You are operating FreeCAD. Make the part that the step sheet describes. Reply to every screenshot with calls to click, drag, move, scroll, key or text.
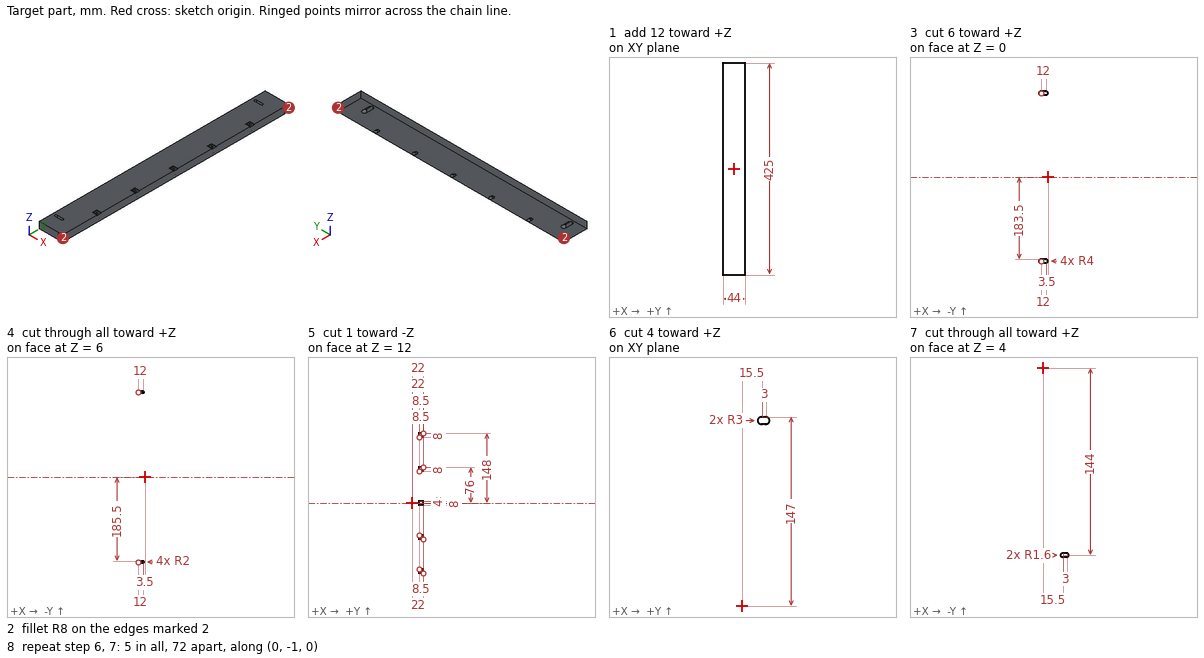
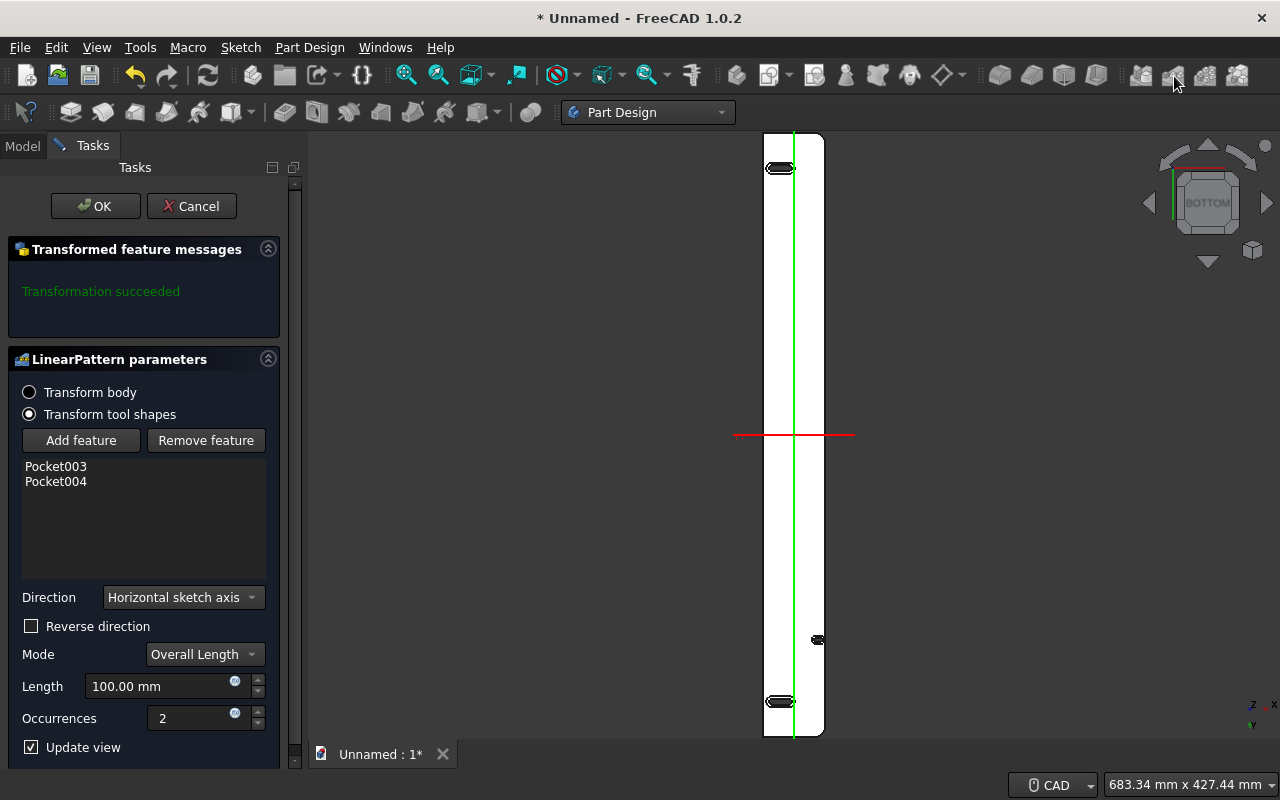
click(184, 598)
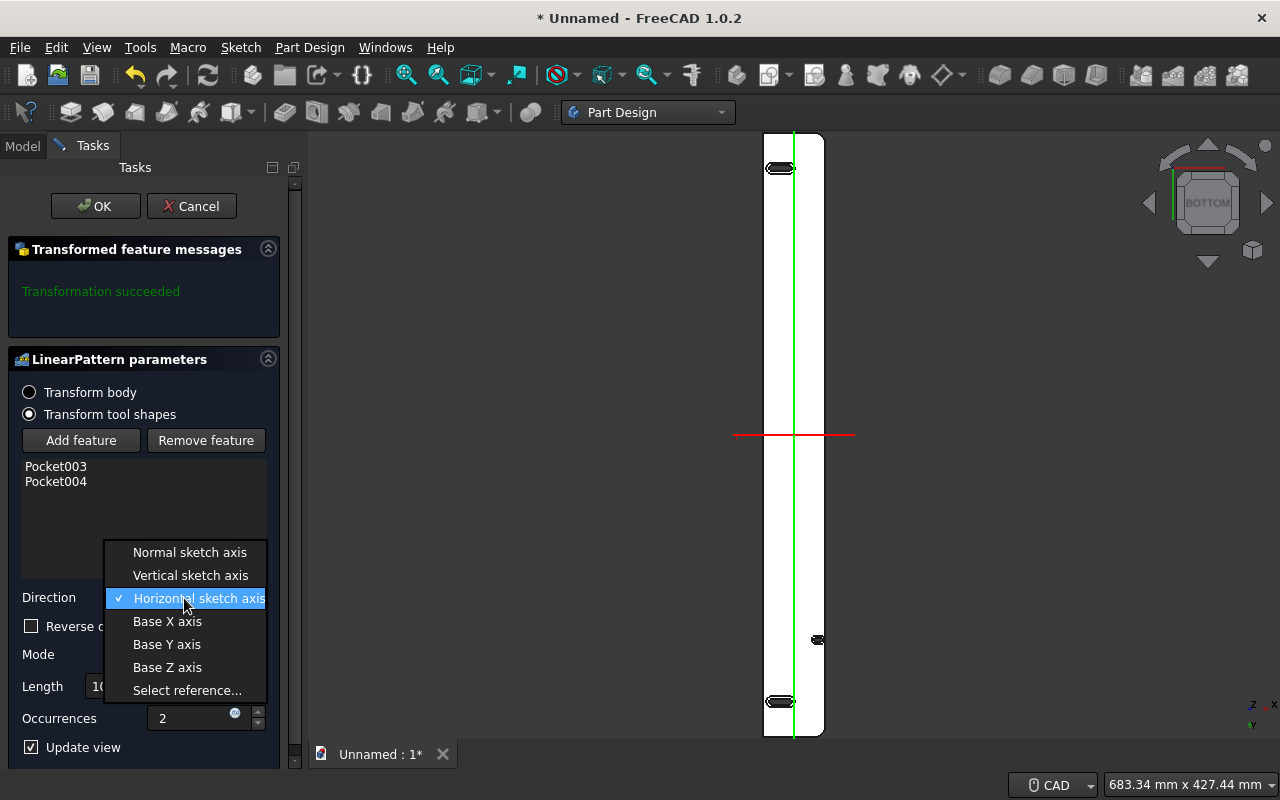
click(184, 644)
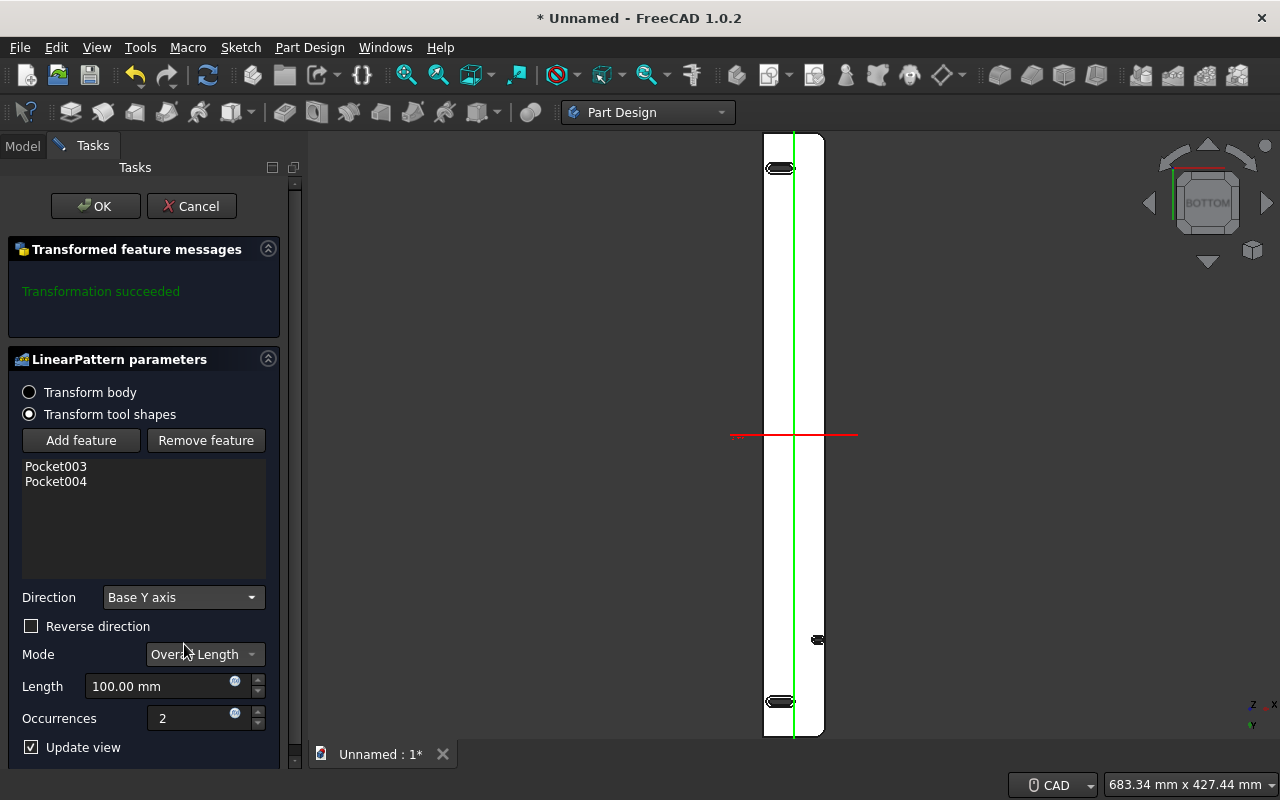
click(206, 654)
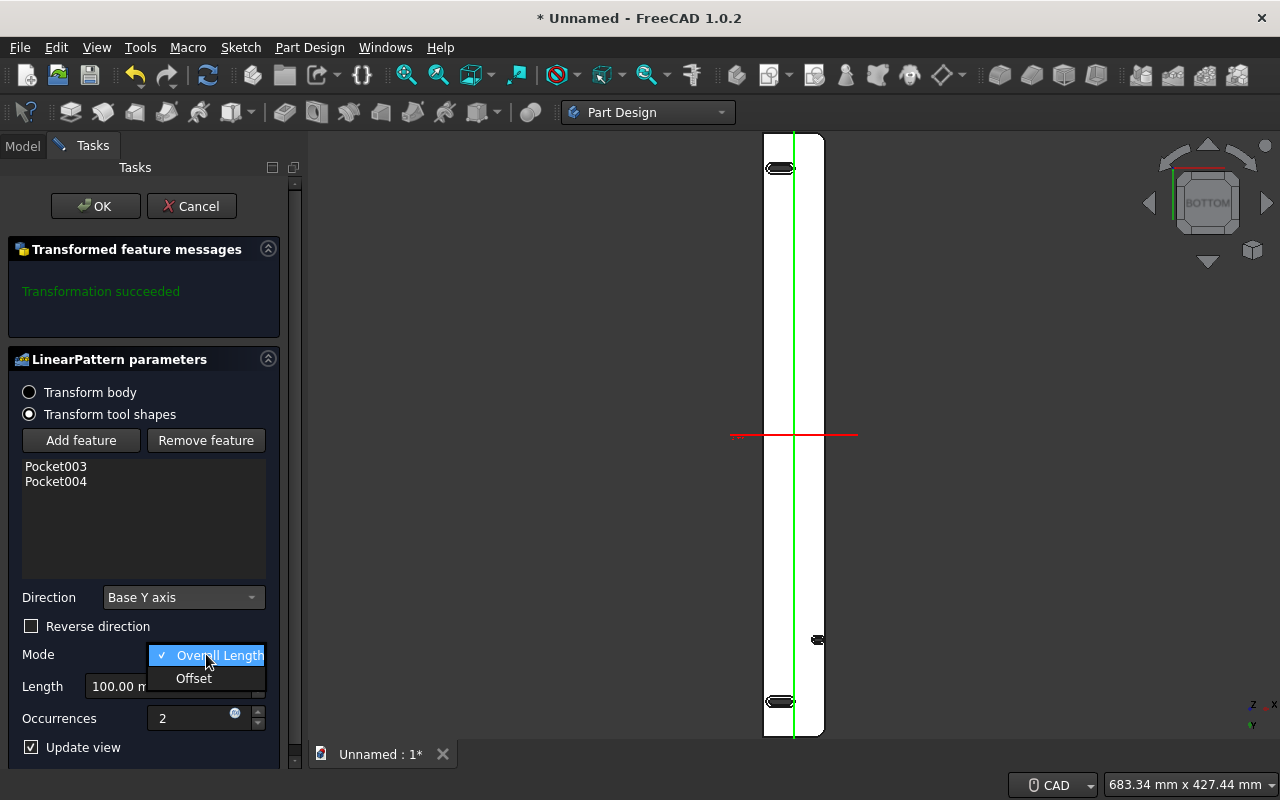
click(206, 678)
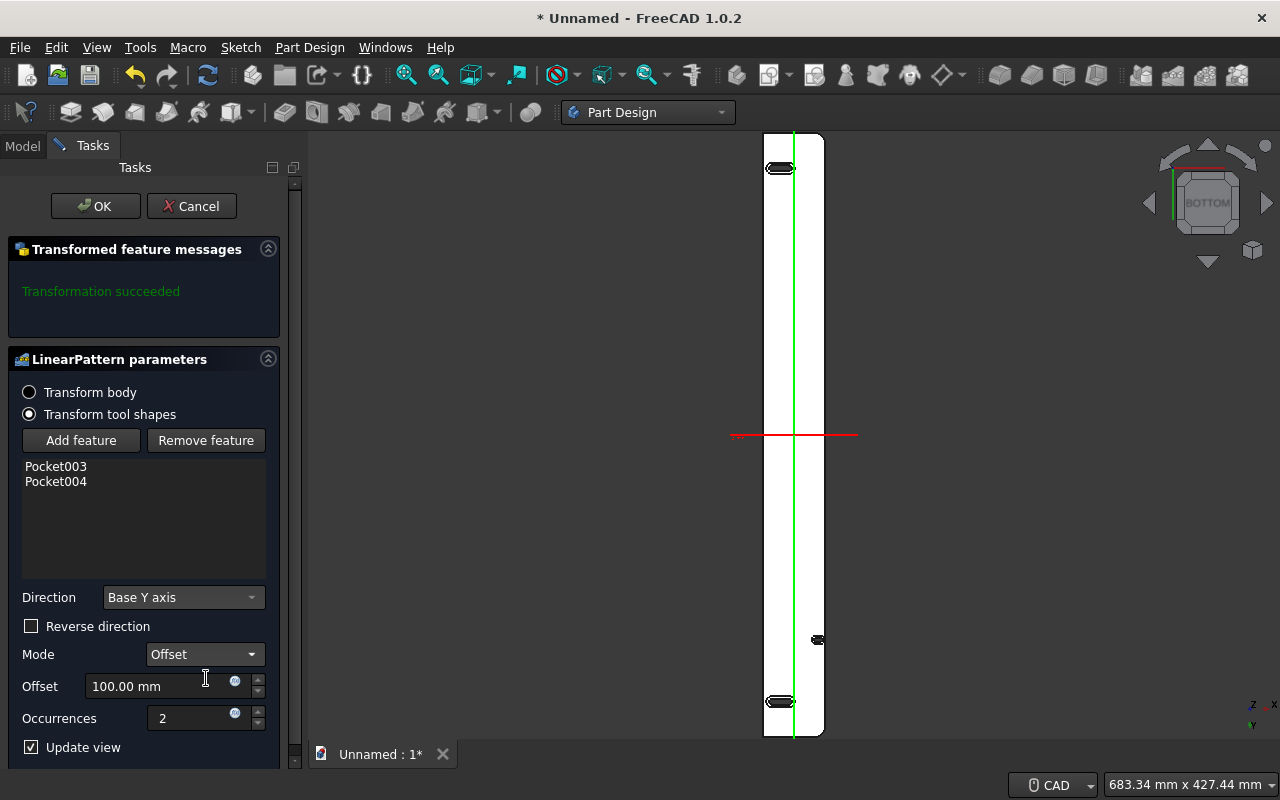
triple_click(168, 686)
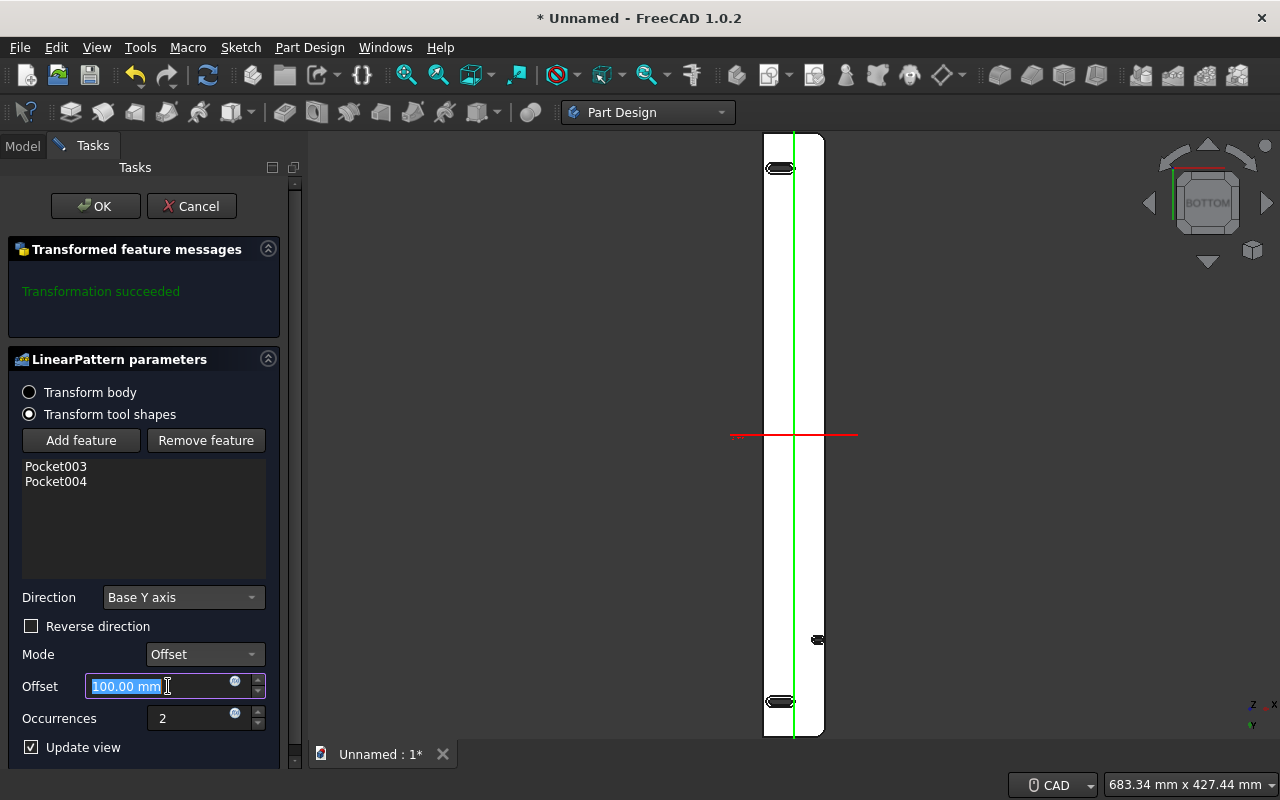
text(72)
key(Tab)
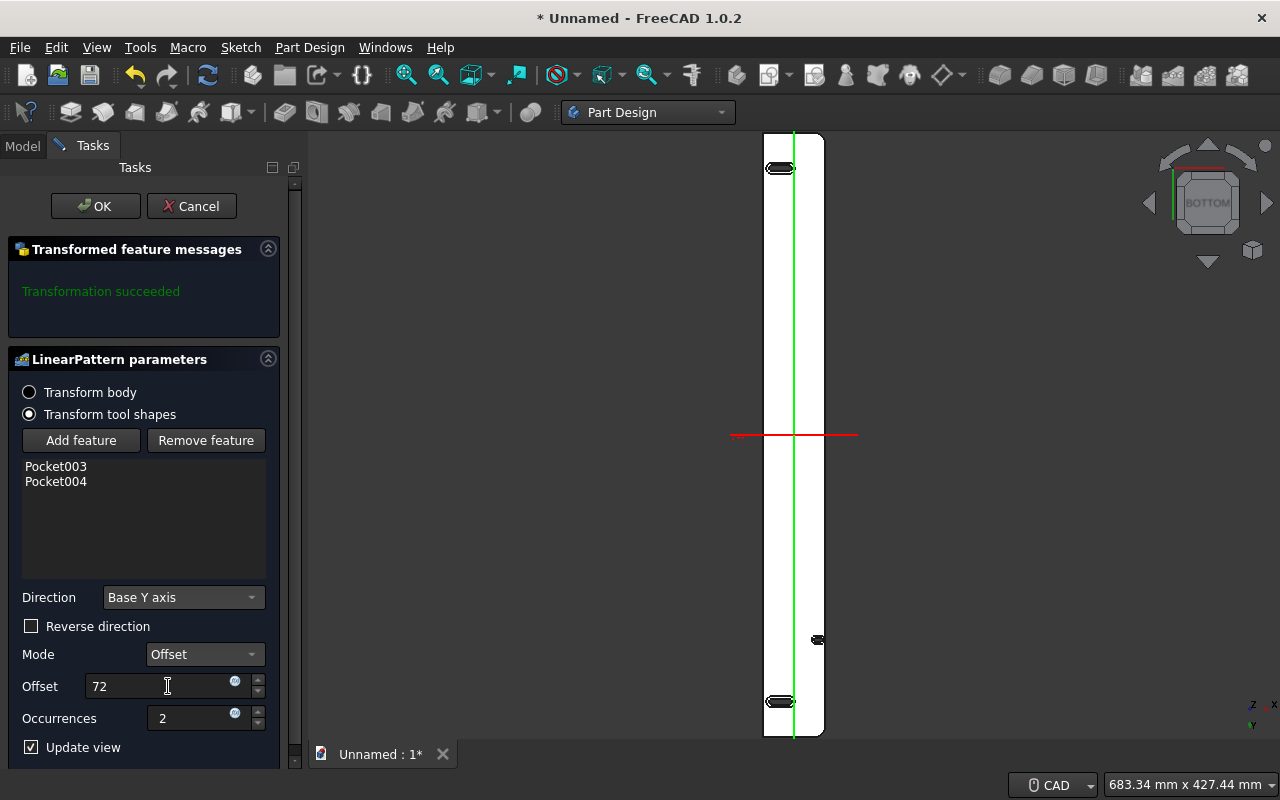
triple_click(198, 718)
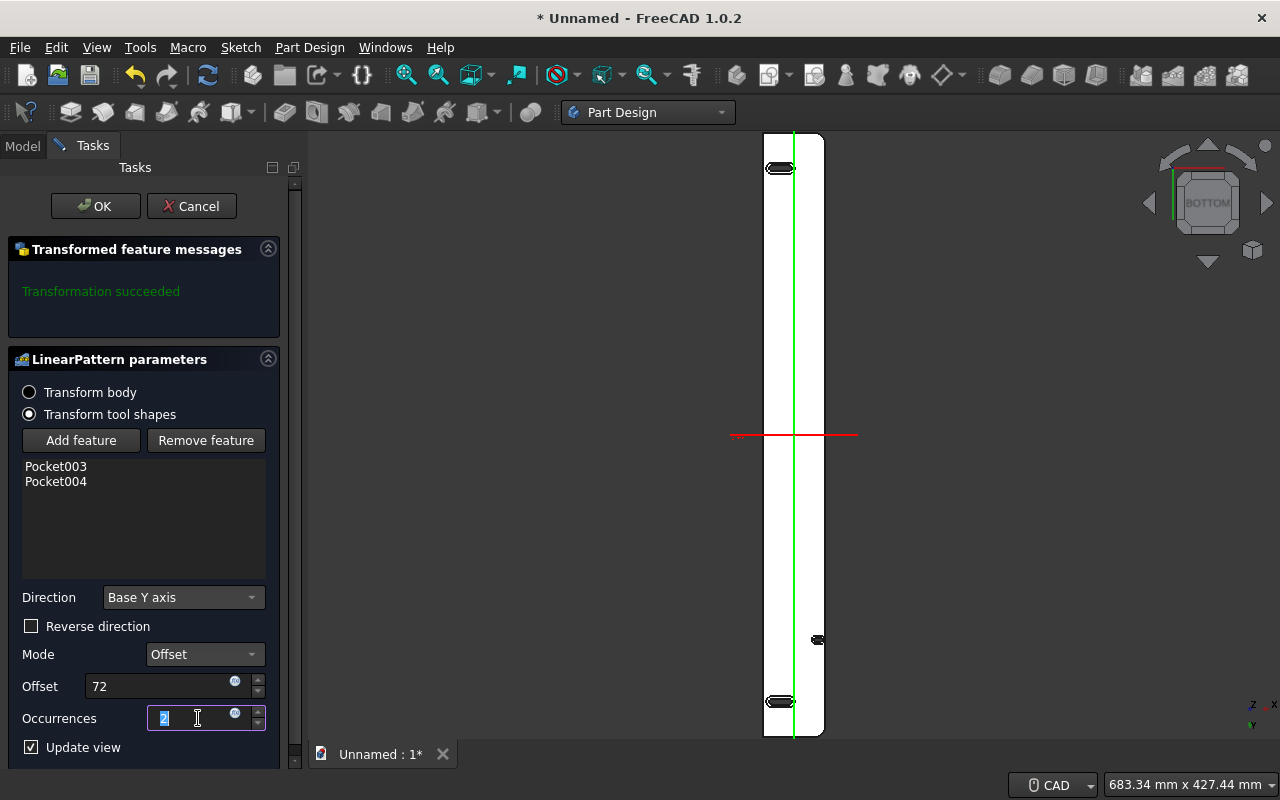
text(5)
key(Tab)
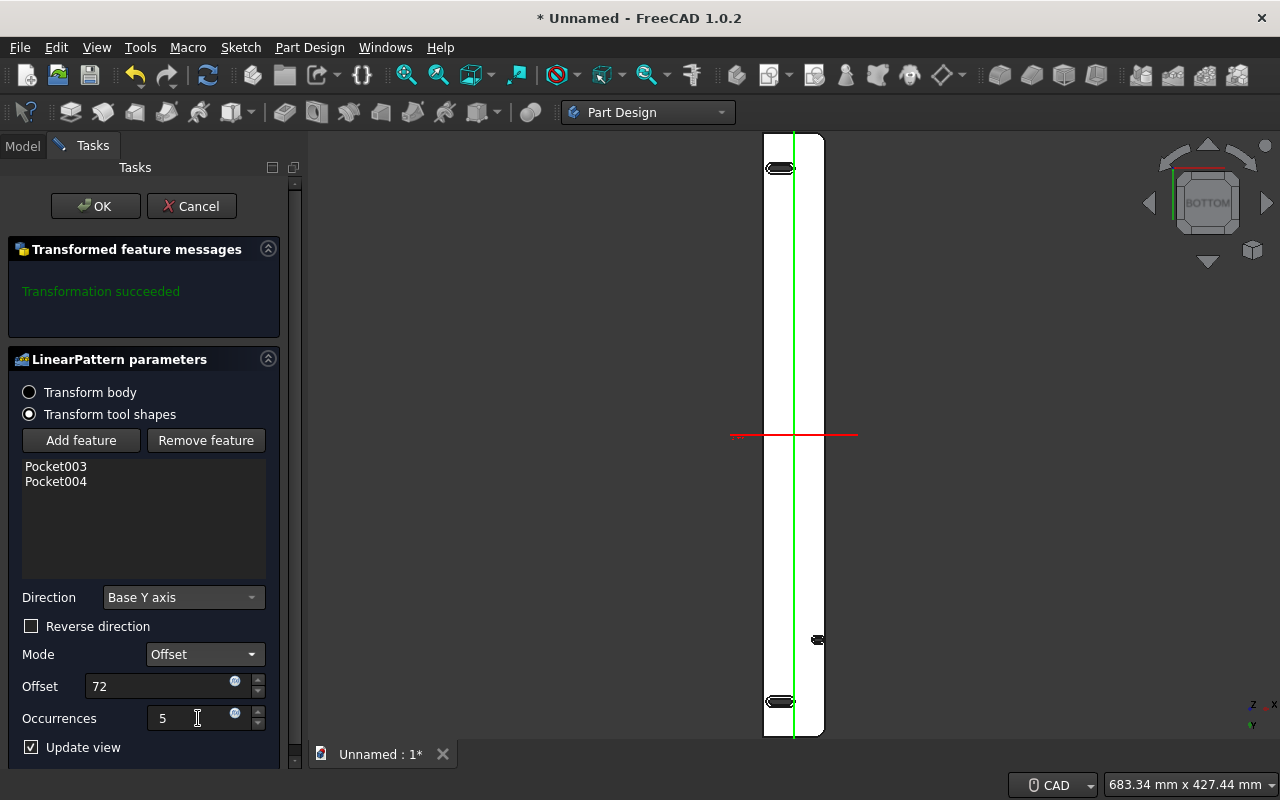
click(30, 626)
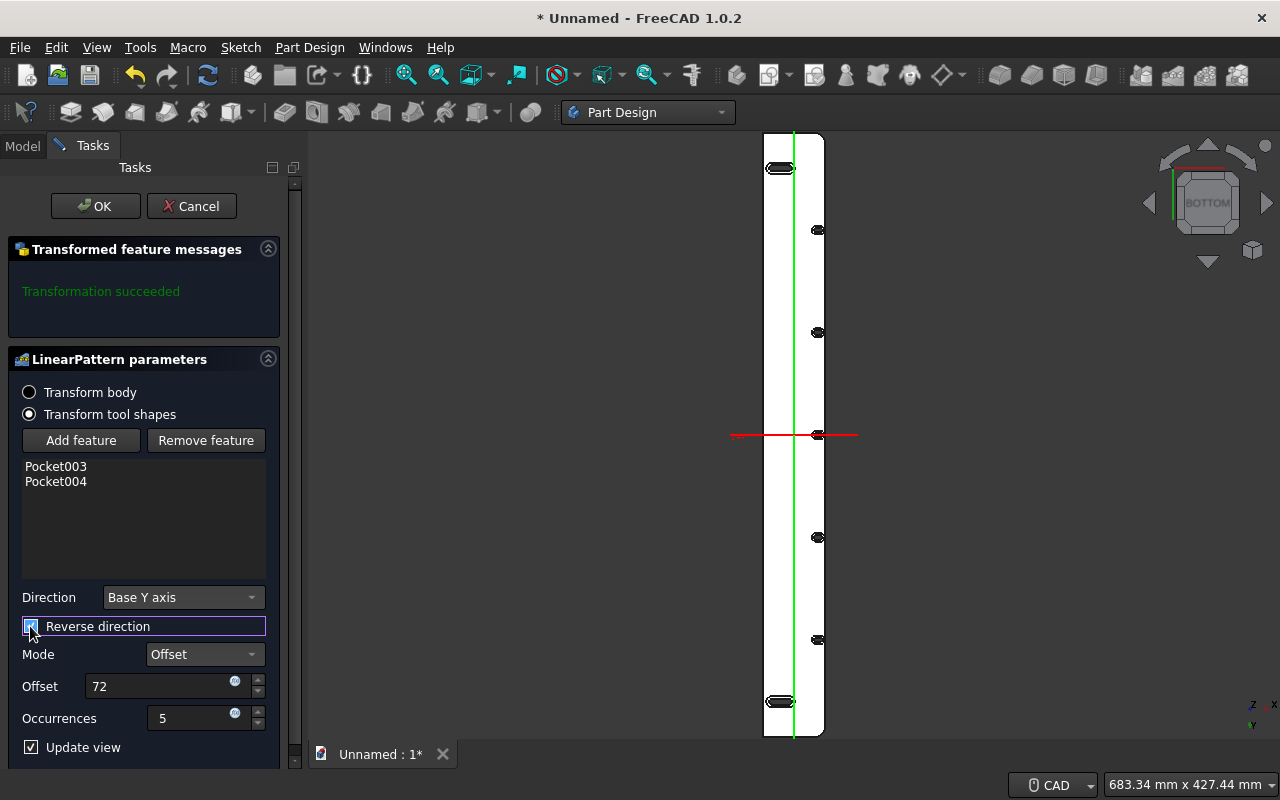
click(96, 206)